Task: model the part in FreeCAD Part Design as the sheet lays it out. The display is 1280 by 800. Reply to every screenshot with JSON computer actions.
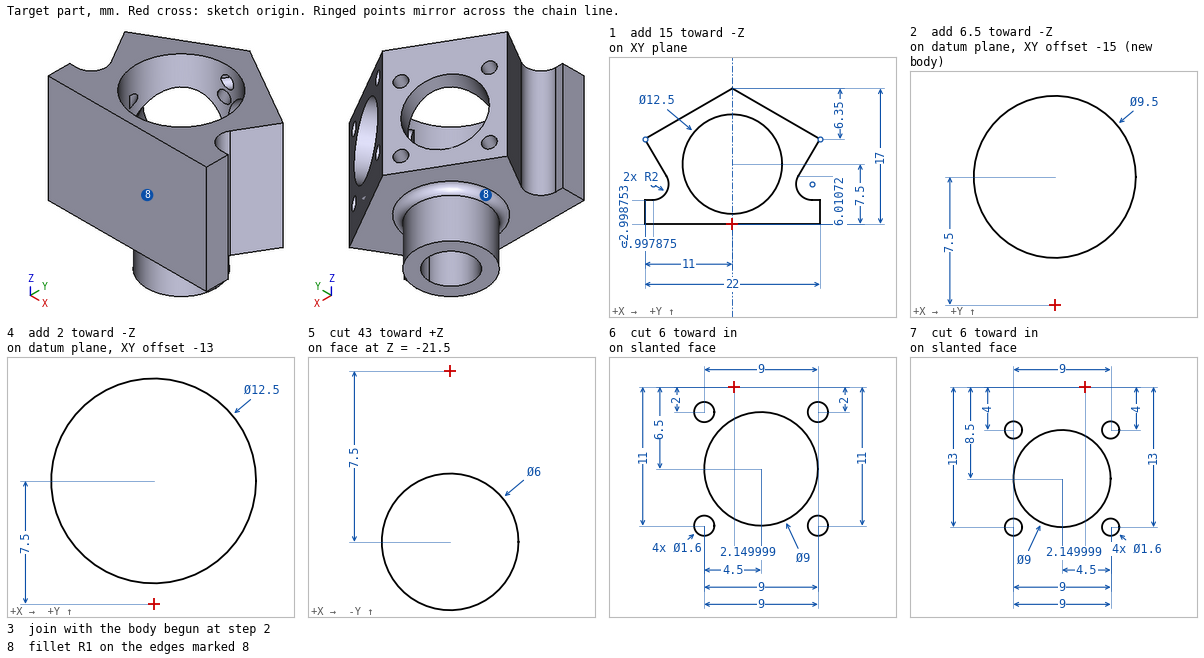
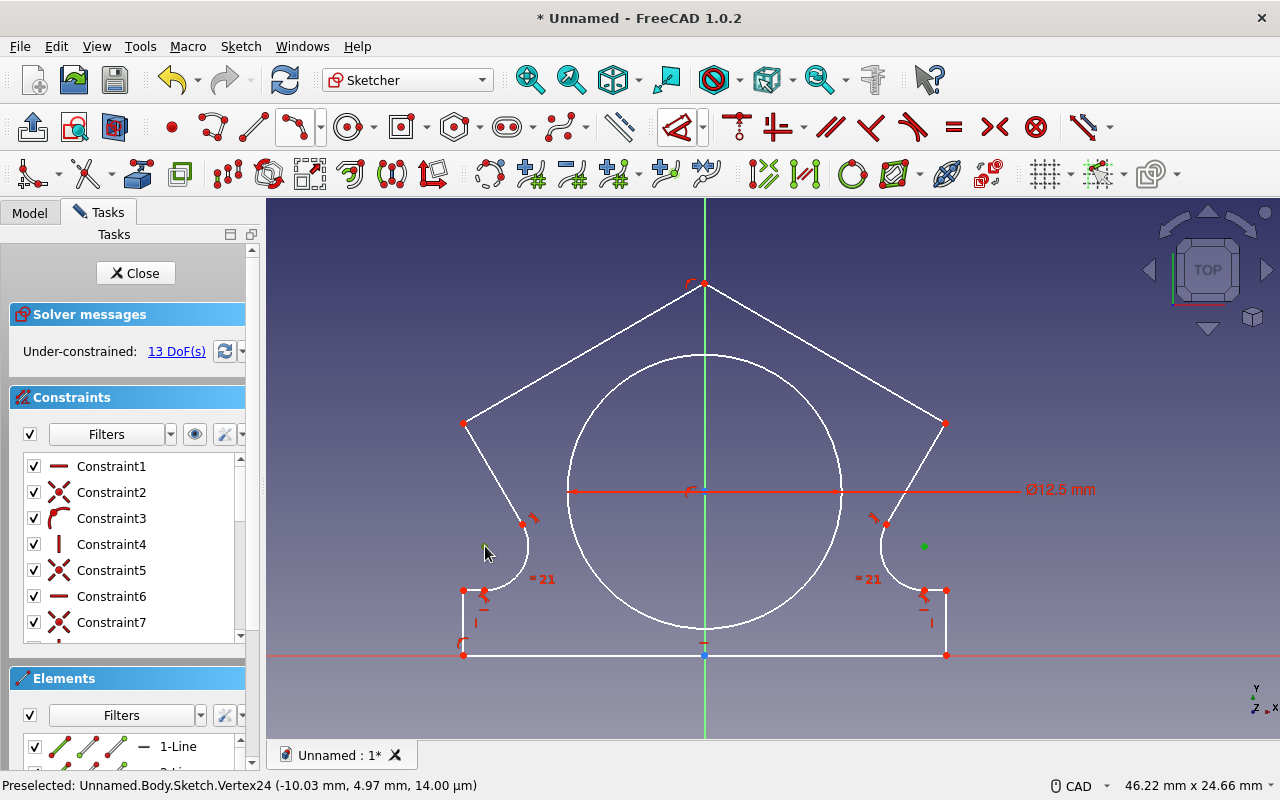
{"action": "left_click", "coordinate": [705, 572]}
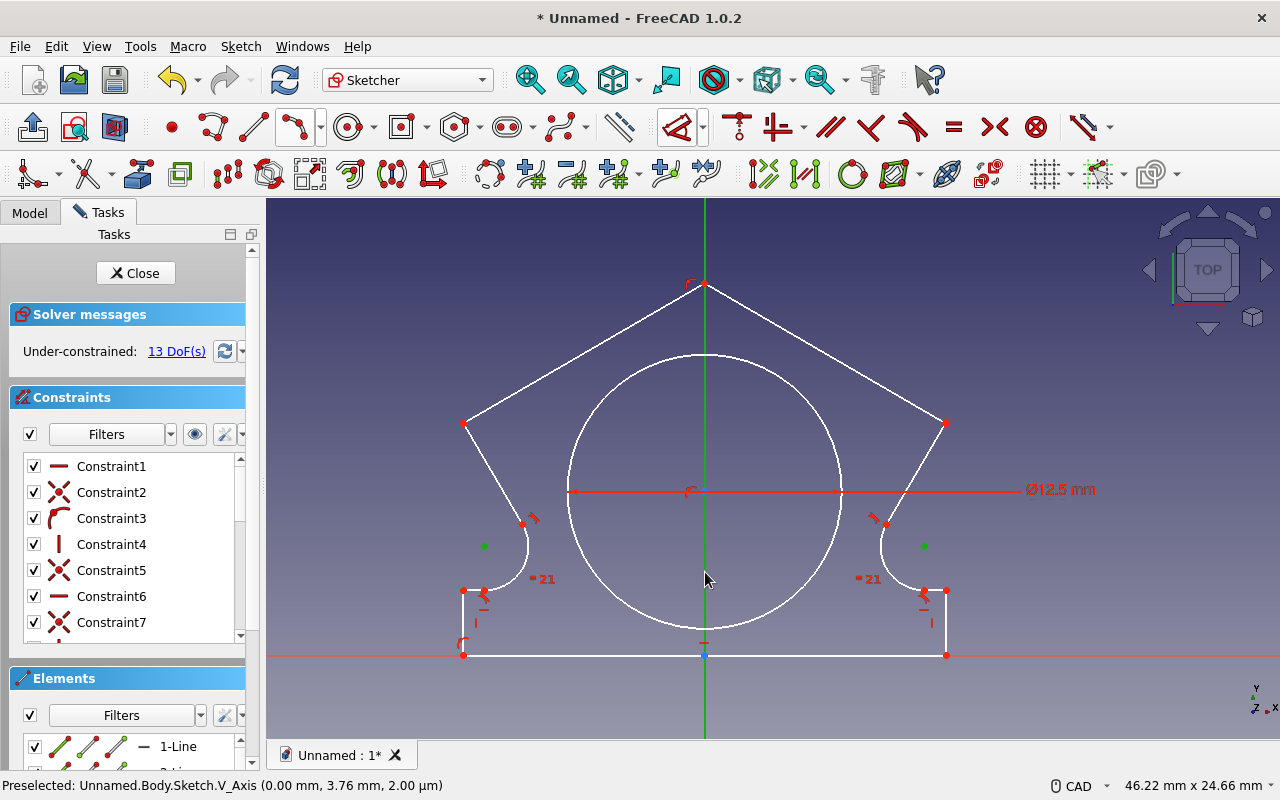
{"action": "left_click", "coordinate": [995, 128]}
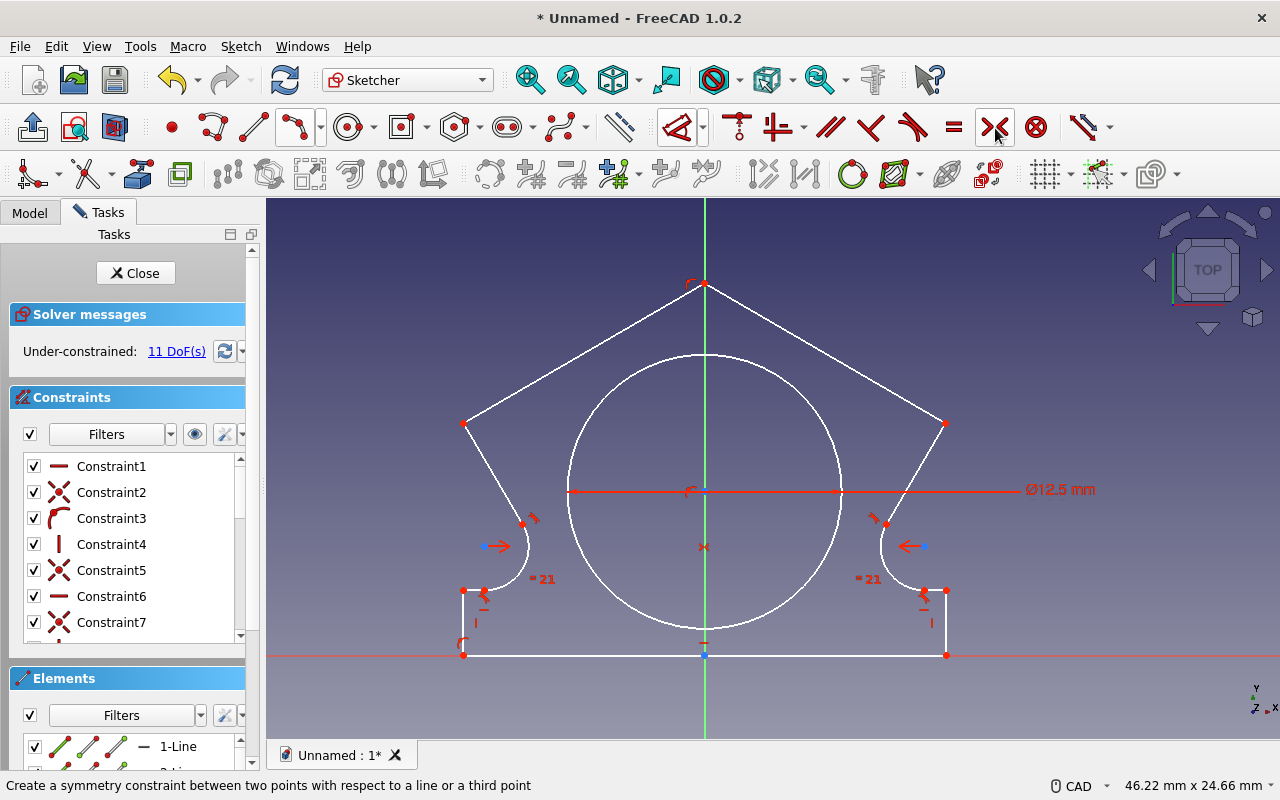
{"action": "left_click", "coordinate": [945, 423]}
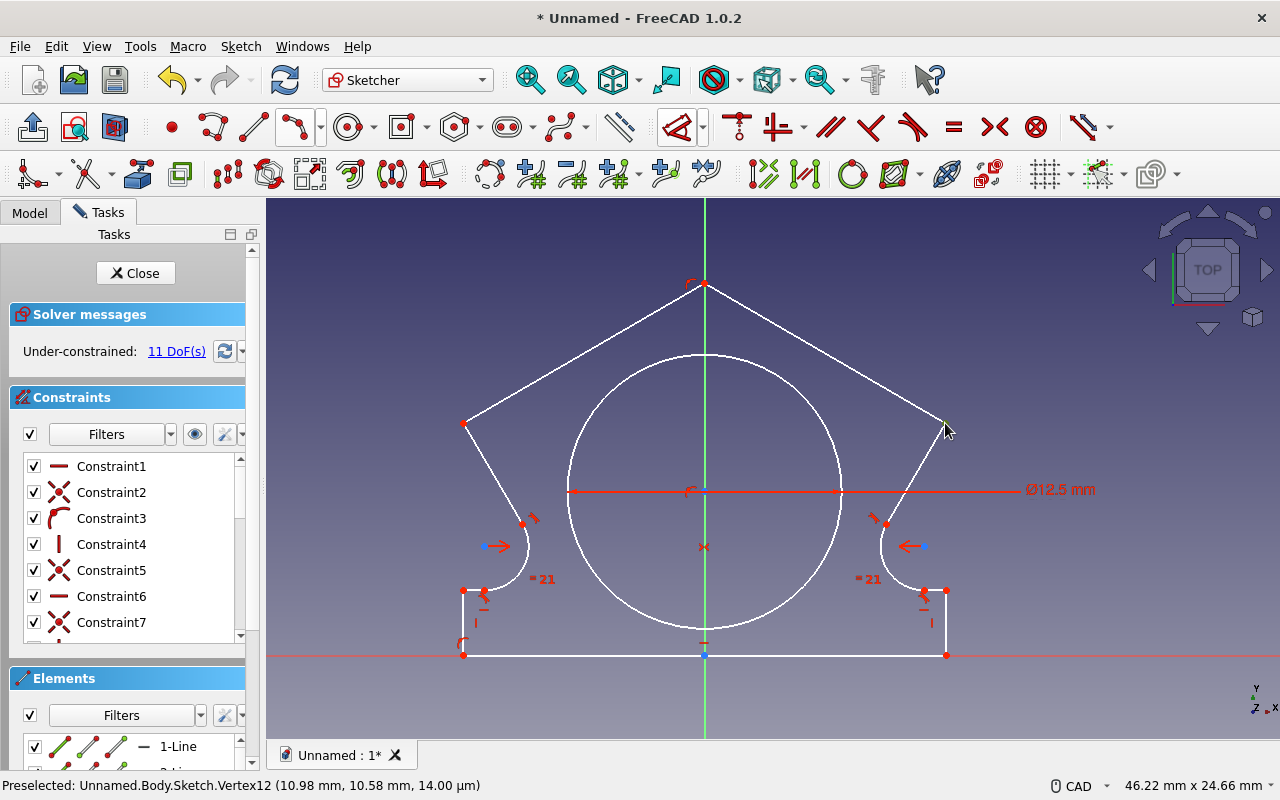
{"action": "left_click", "coordinate": [463, 423]}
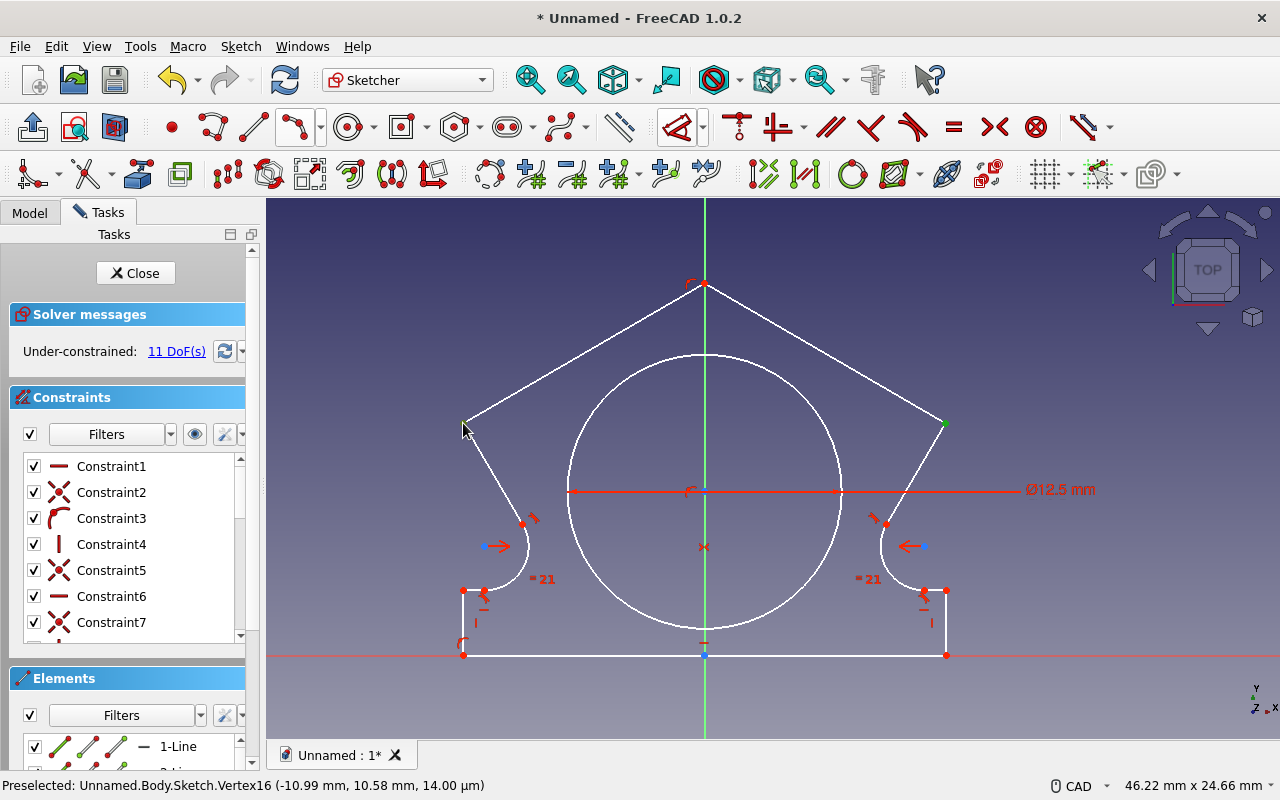
{"action": "left_click", "coordinate": [705, 572]}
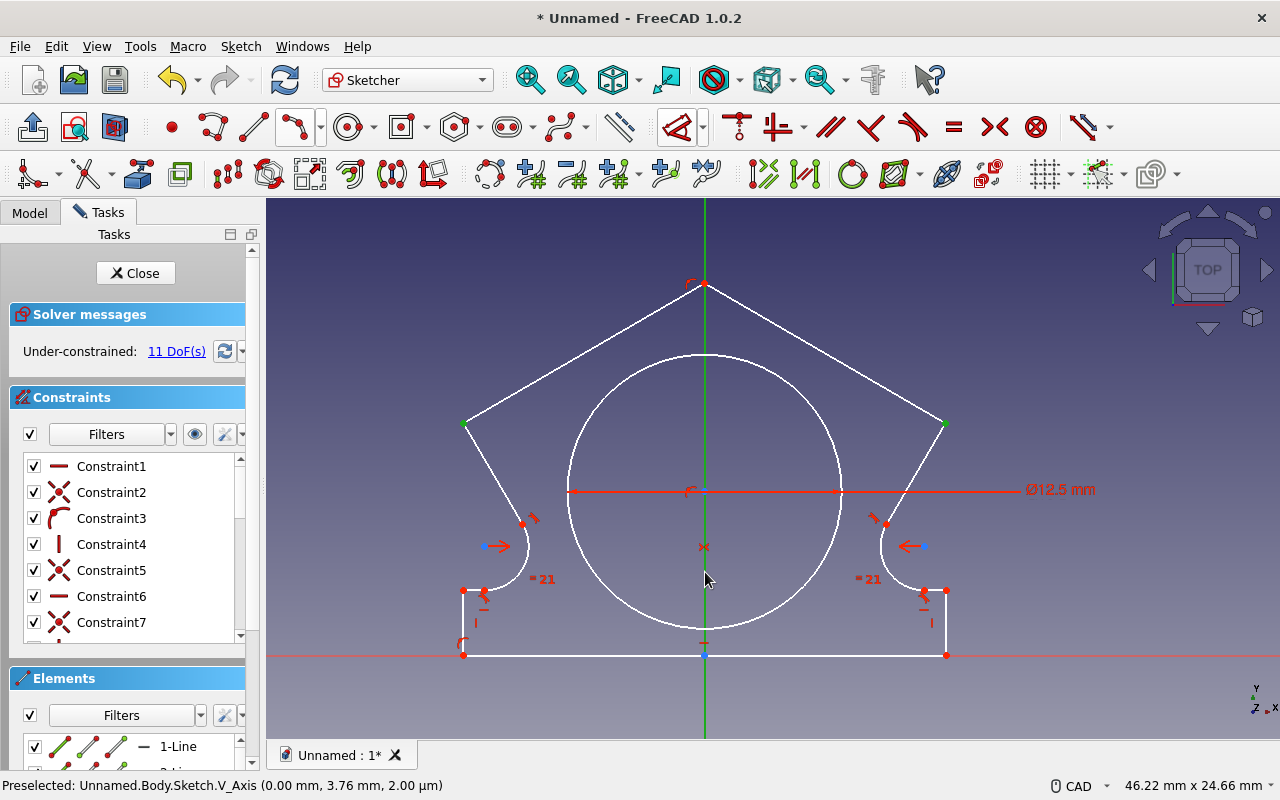
{"action": "left_click", "coordinate": [995, 128]}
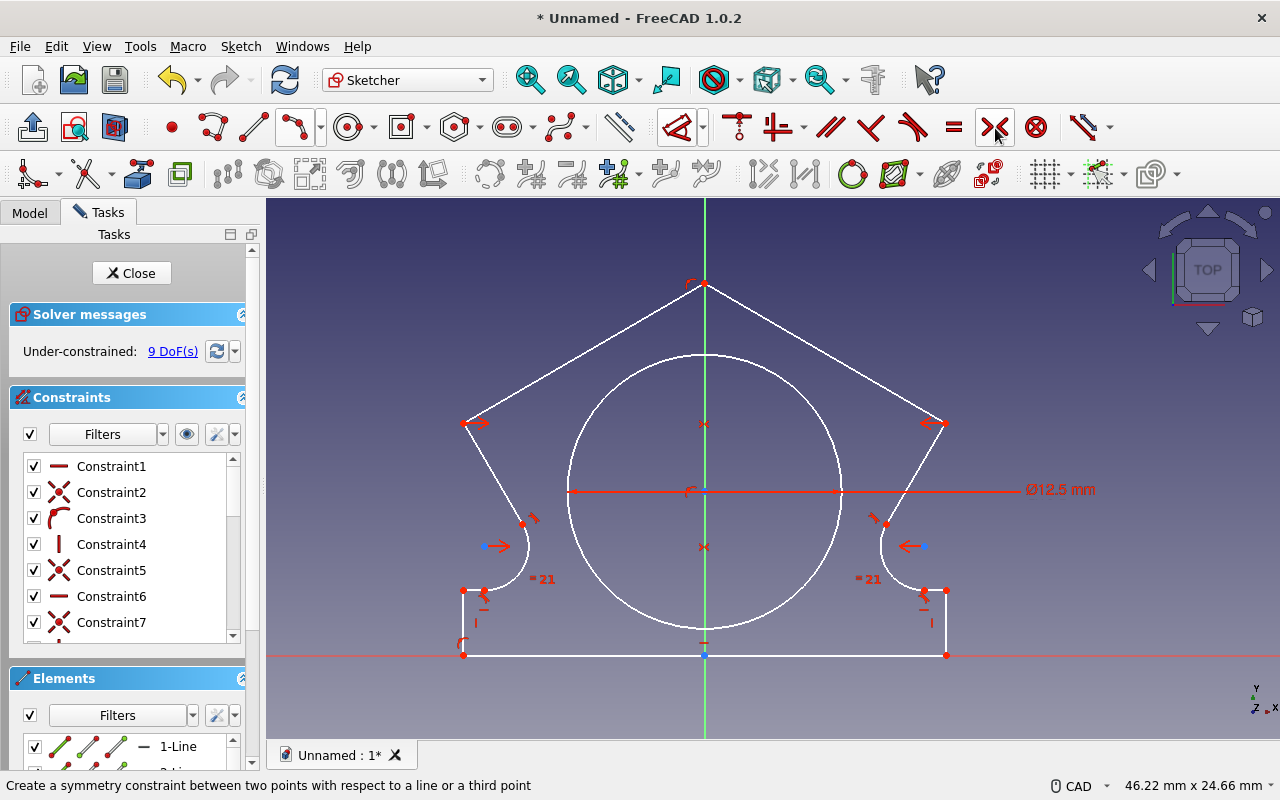
{"action": "left_click", "coordinate": [676, 128]}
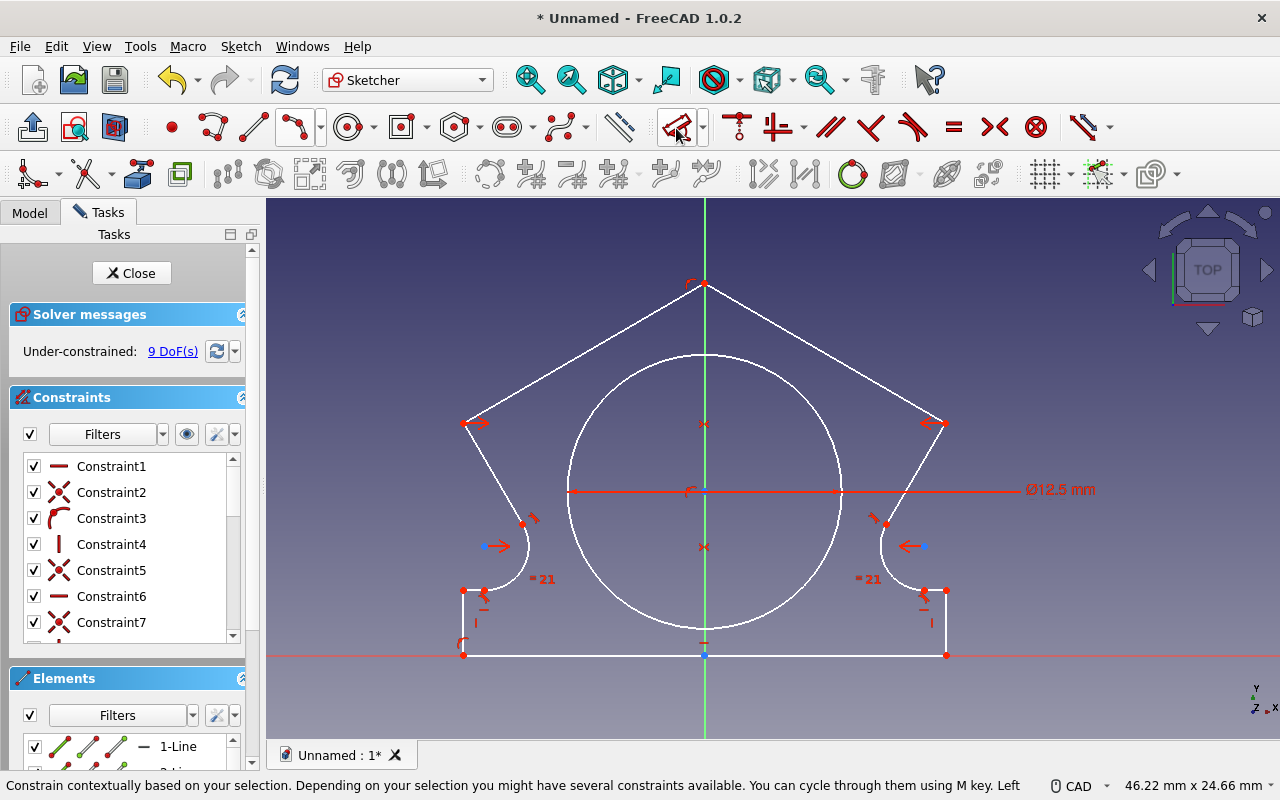
{"action": "left_click", "coordinate": [881, 551]}
{"action": "left_click", "coordinate": [849, 554]}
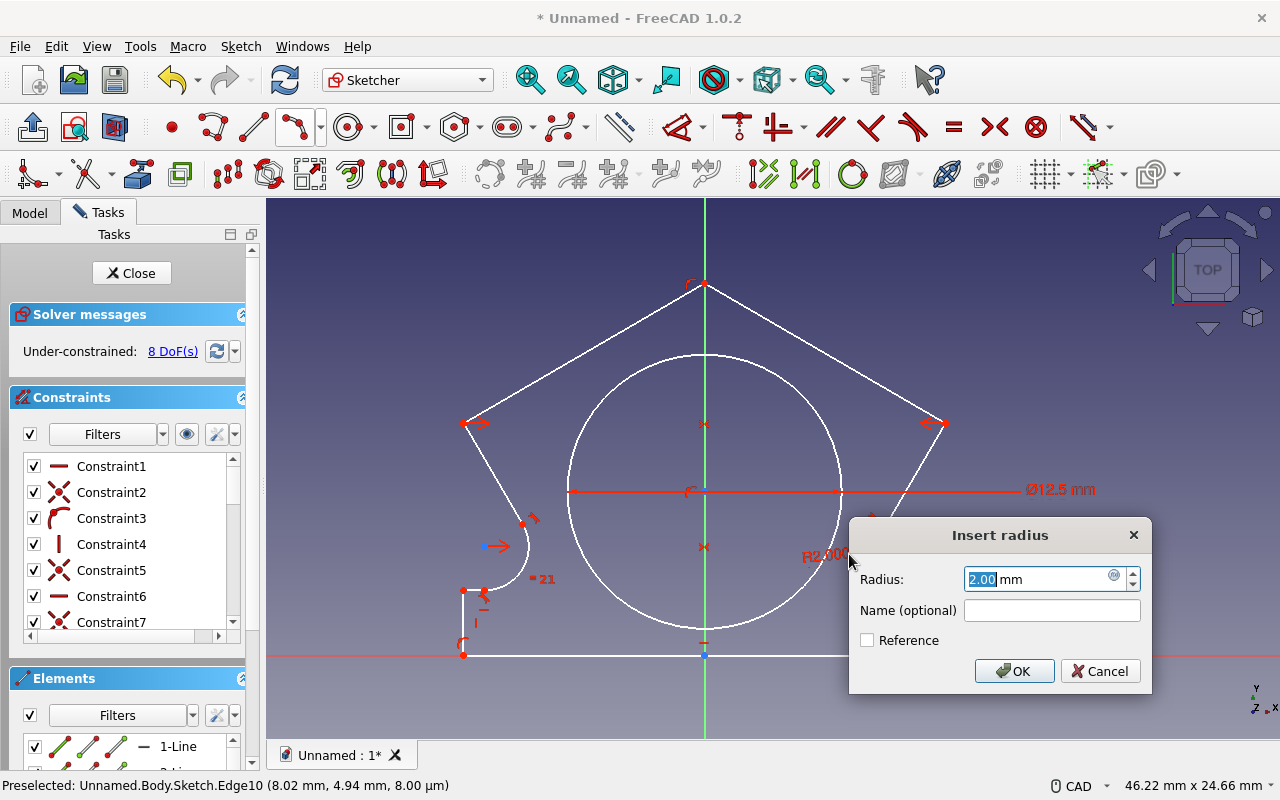
{"action": "type", "text": "2"}
{"action": "key", "text": "Return"}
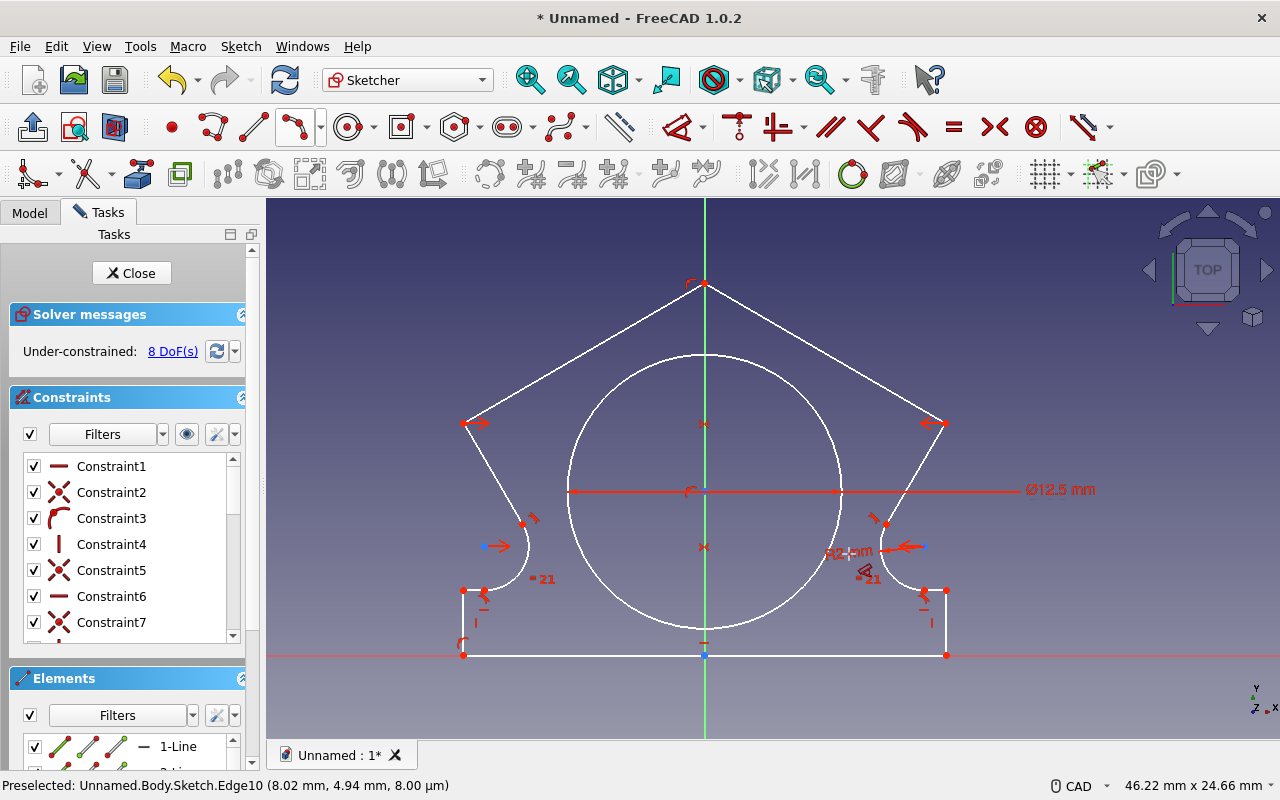
{"action": "left_click", "coordinate": [608, 656]}
{"action": "left_click", "coordinate": [594, 690]}